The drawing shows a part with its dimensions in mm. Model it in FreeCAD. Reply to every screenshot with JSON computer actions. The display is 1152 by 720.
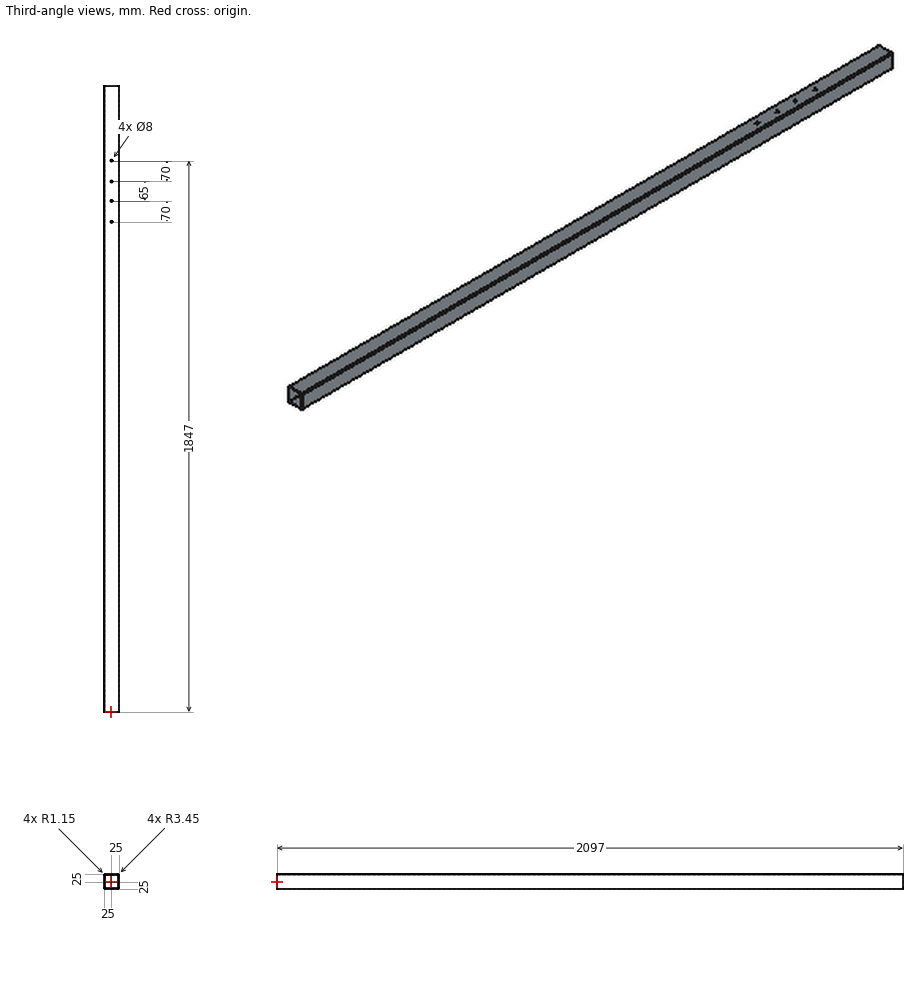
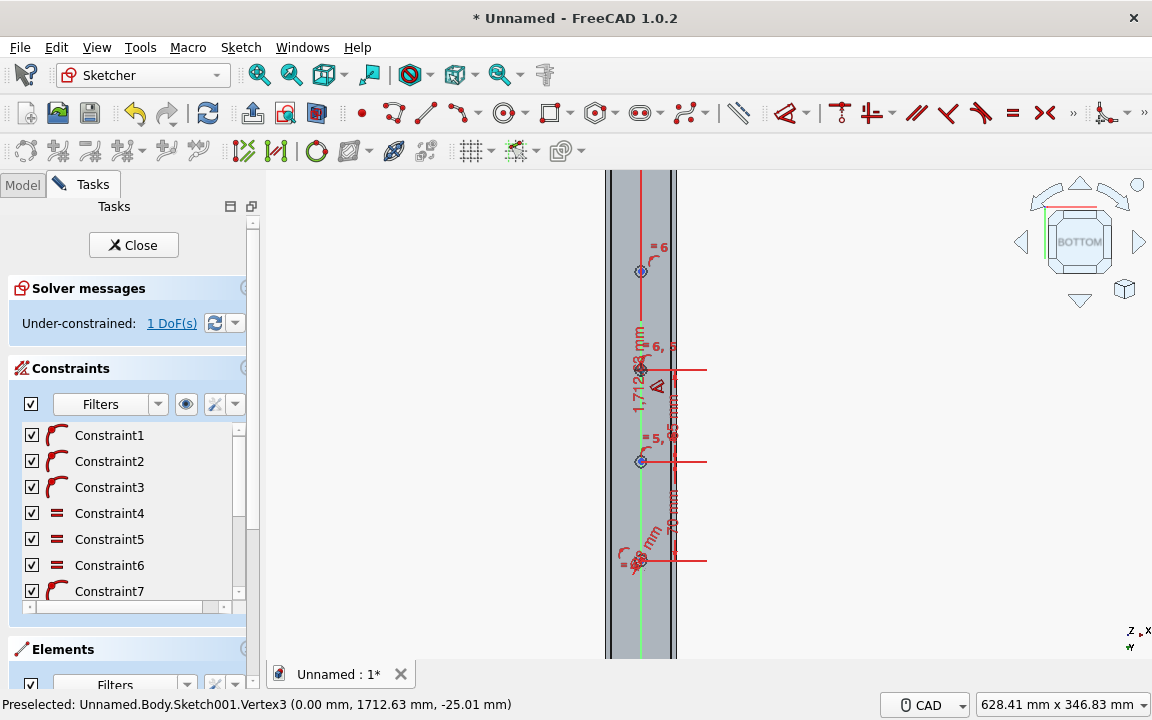
{"action": "left_click", "coordinate": [641, 272]}
{"action": "left_click", "coordinate": [675, 321]}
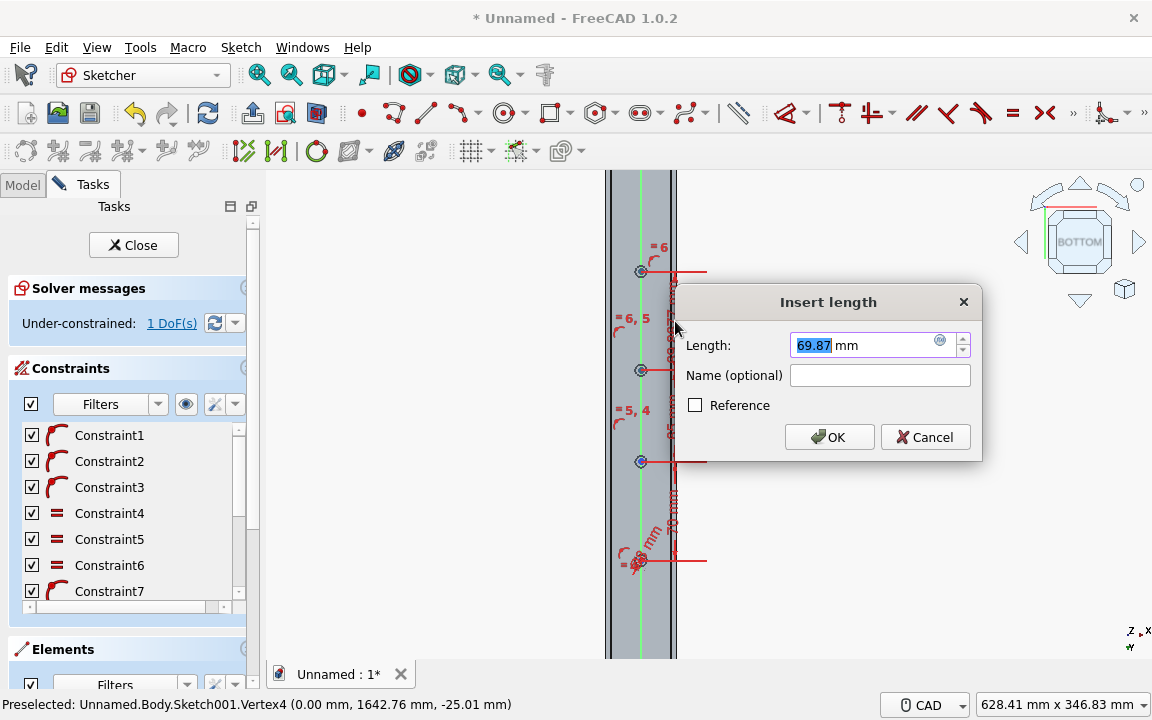
{"action": "type", "text": "70"}
{"action": "key", "text": "Return"}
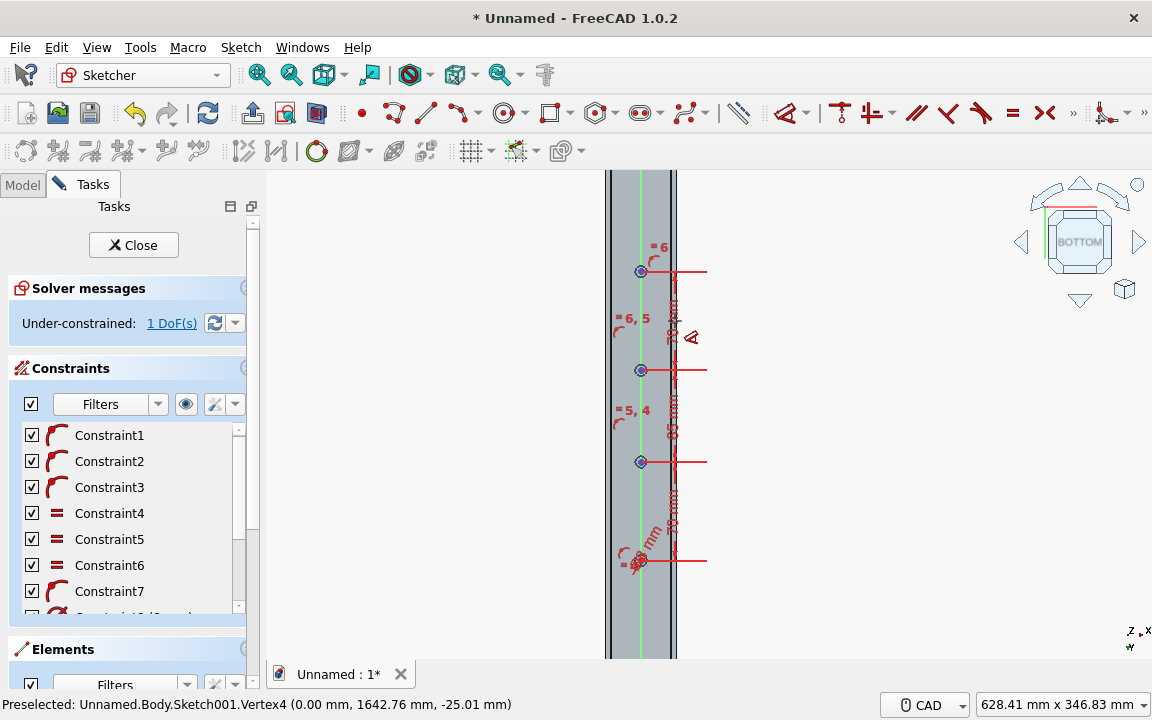
{"action": "left_click", "coordinate": [641, 561]}
{"action": "left_click", "coordinate": [675, 379]}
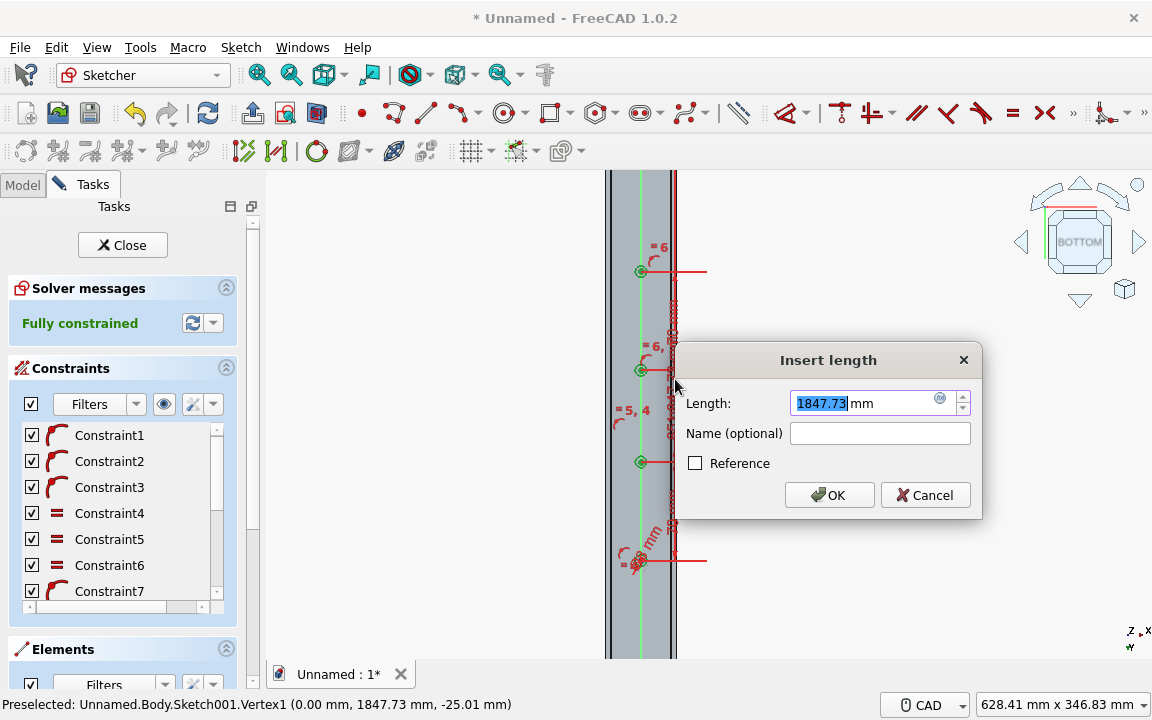
{"action": "type", "text": "1847"}
{"action": "key", "text": "Return"}
{"action": "key", "text": "Escape"}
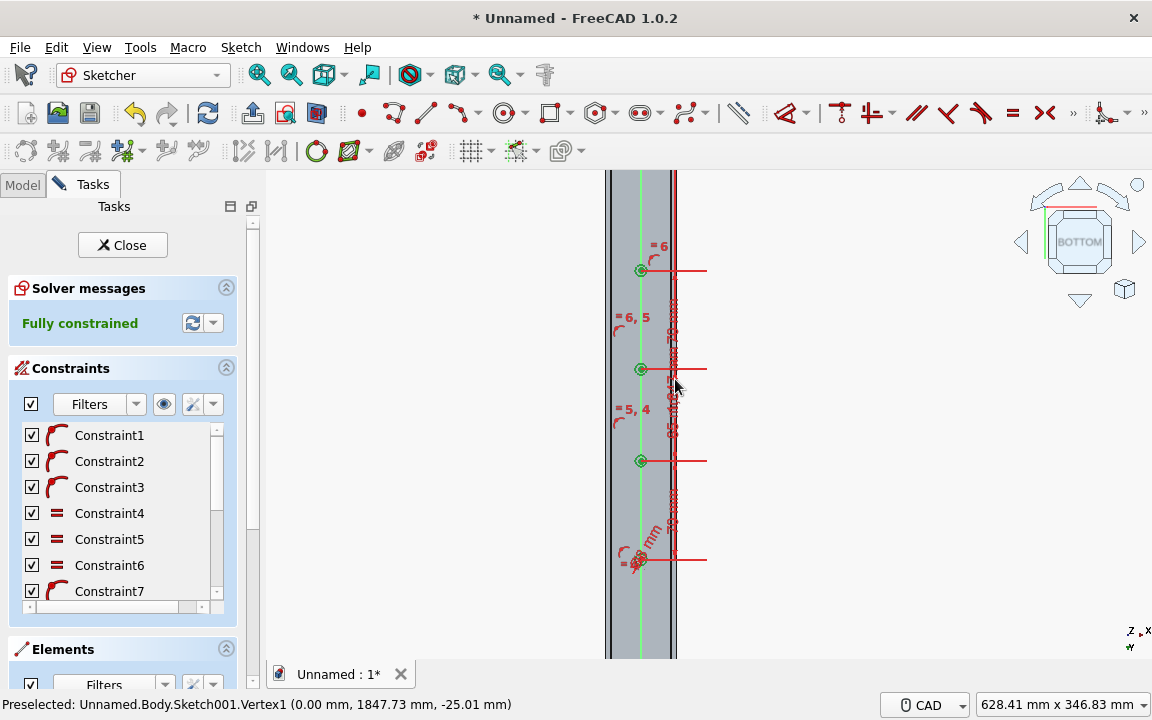
{"action": "left_click", "coordinate": [123, 245]}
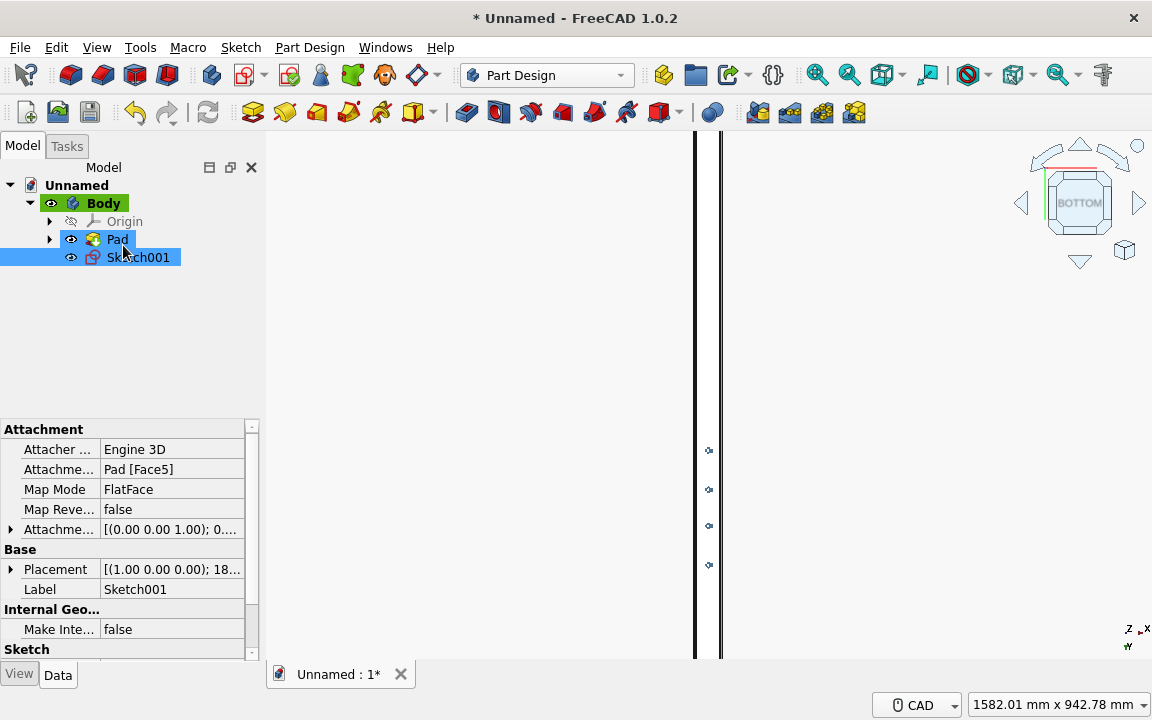
{"action": "left_click", "coordinate": [468, 112]}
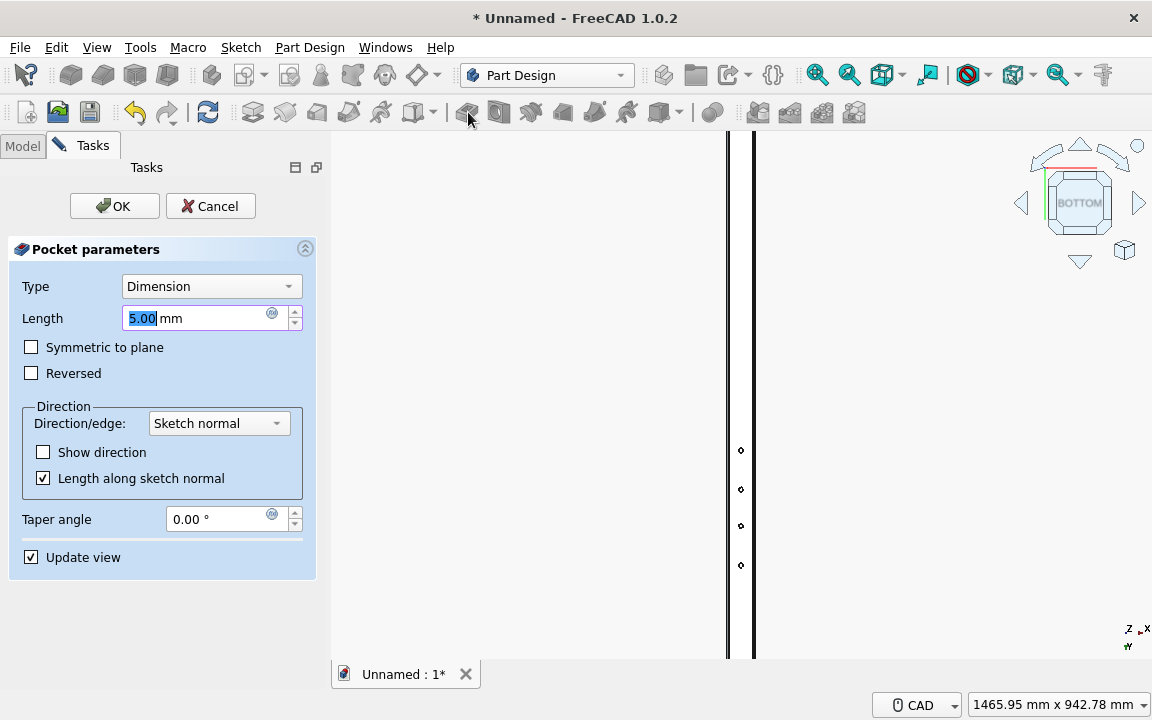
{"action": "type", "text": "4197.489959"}
{"action": "key", "text": "Tab"}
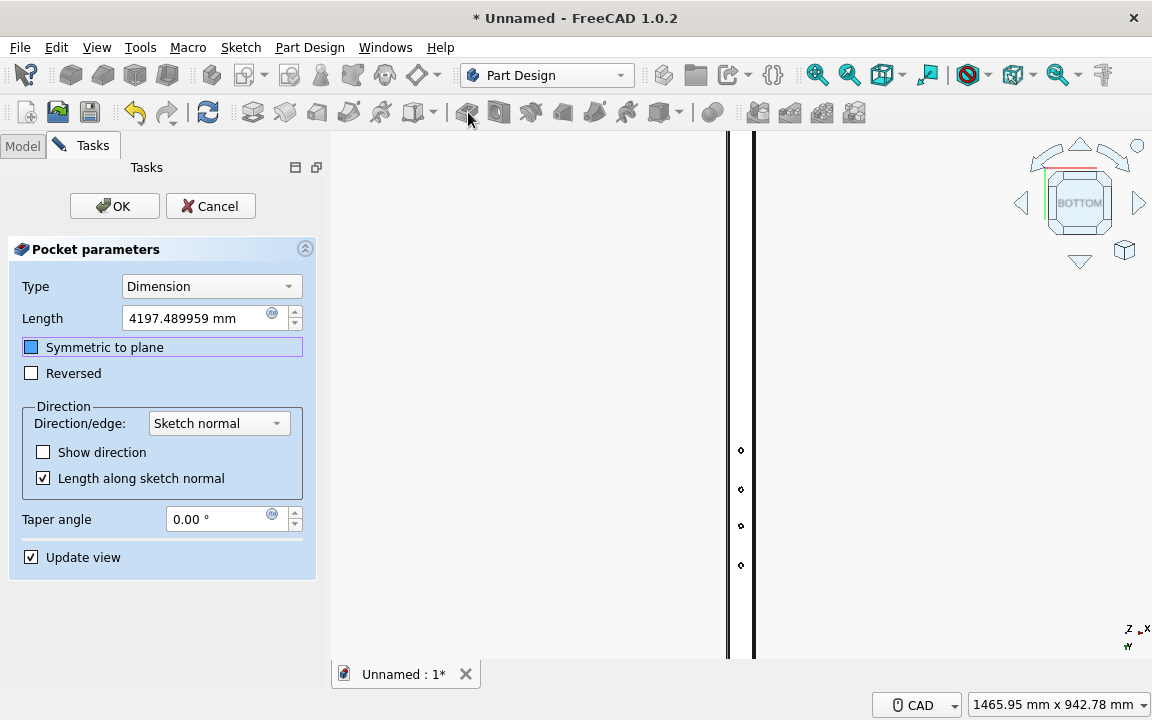
{"action": "left_click", "coordinate": [30, 347]}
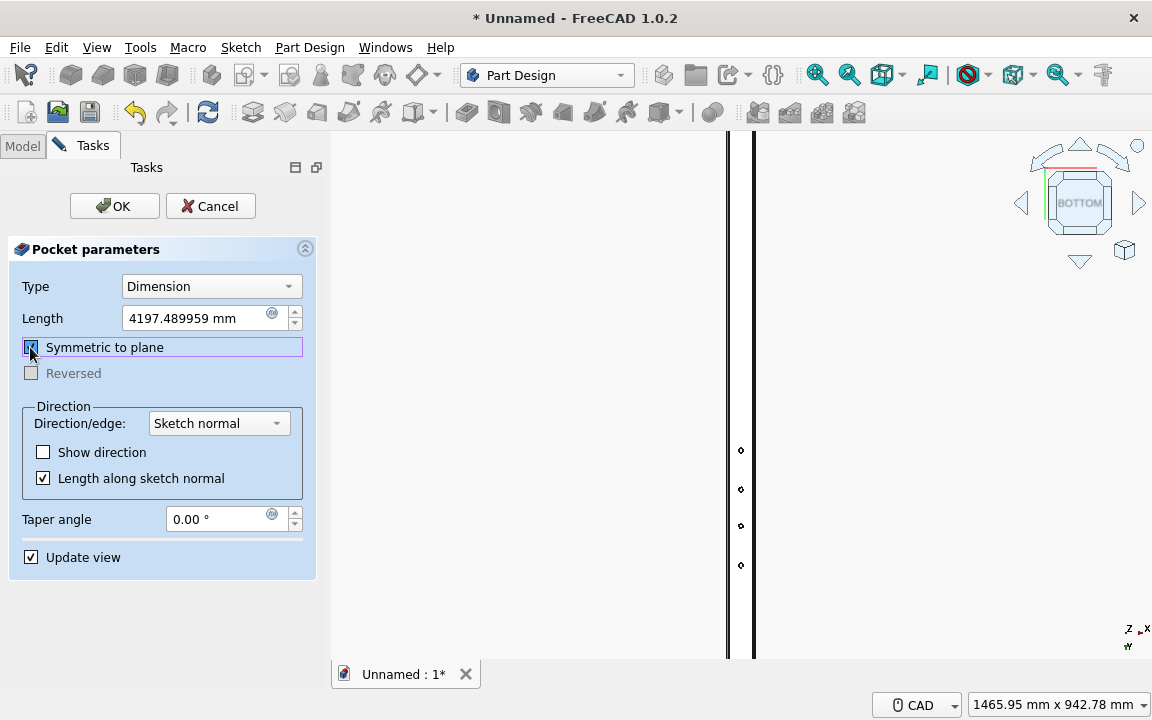
{"action": "left_click", "coordinate": [115, 206]}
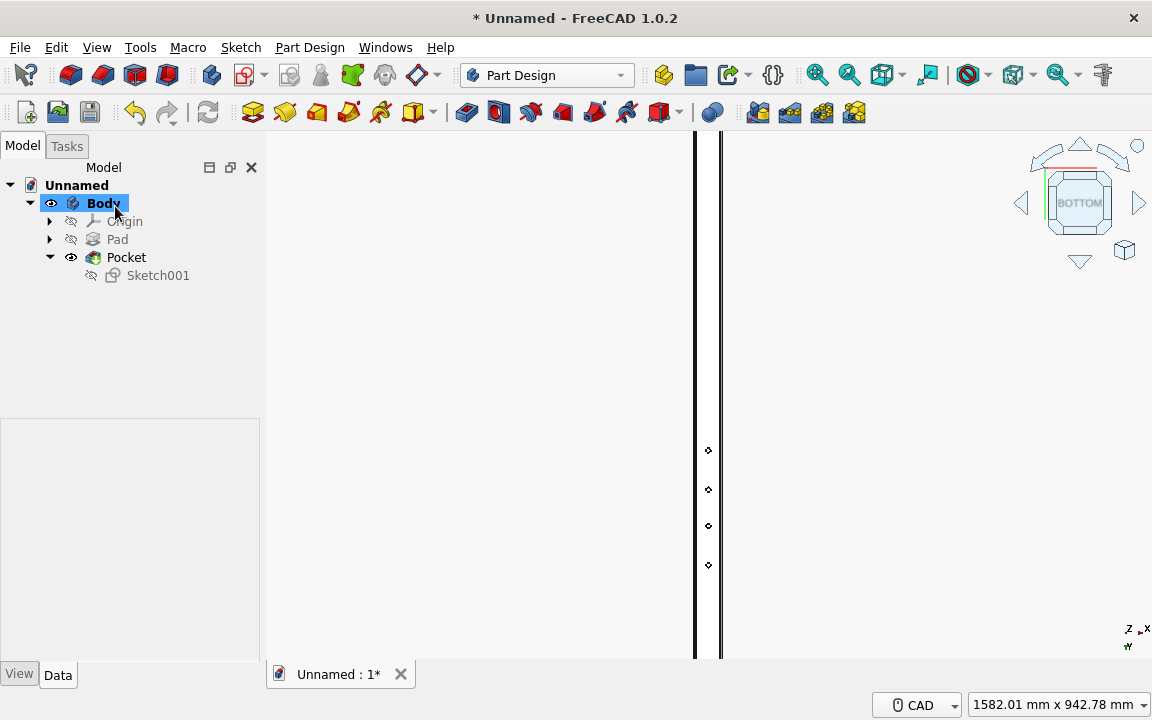
{"action": "key", "text": "0"}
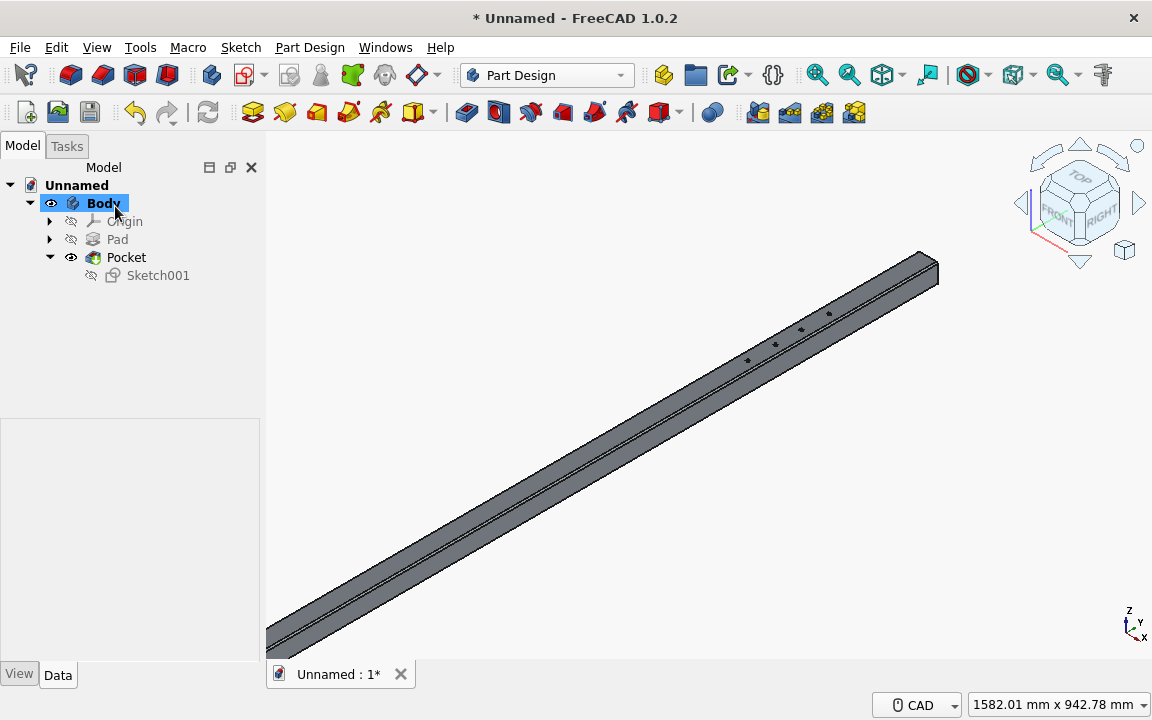
{"action": "left_click", "coordinate": [818, 76]}